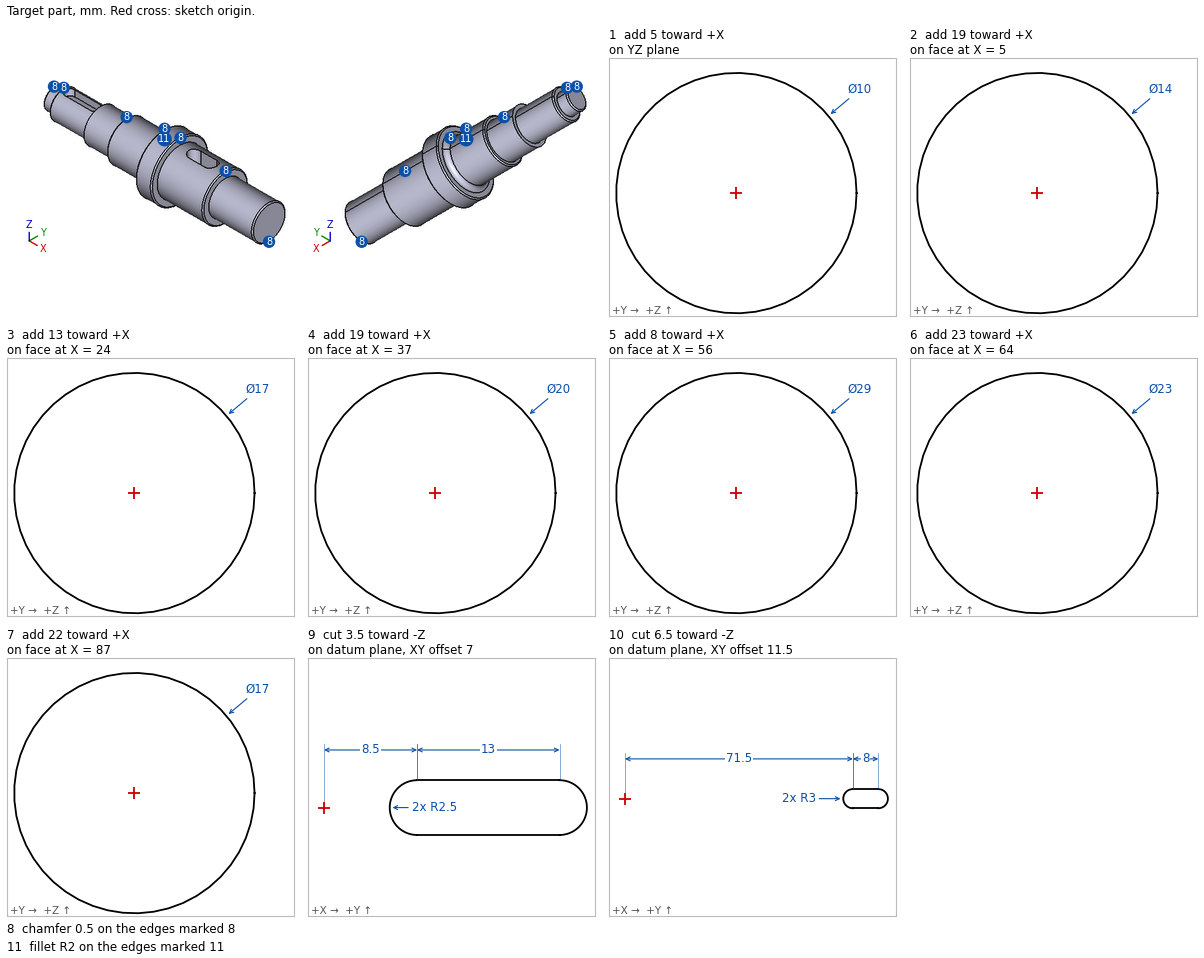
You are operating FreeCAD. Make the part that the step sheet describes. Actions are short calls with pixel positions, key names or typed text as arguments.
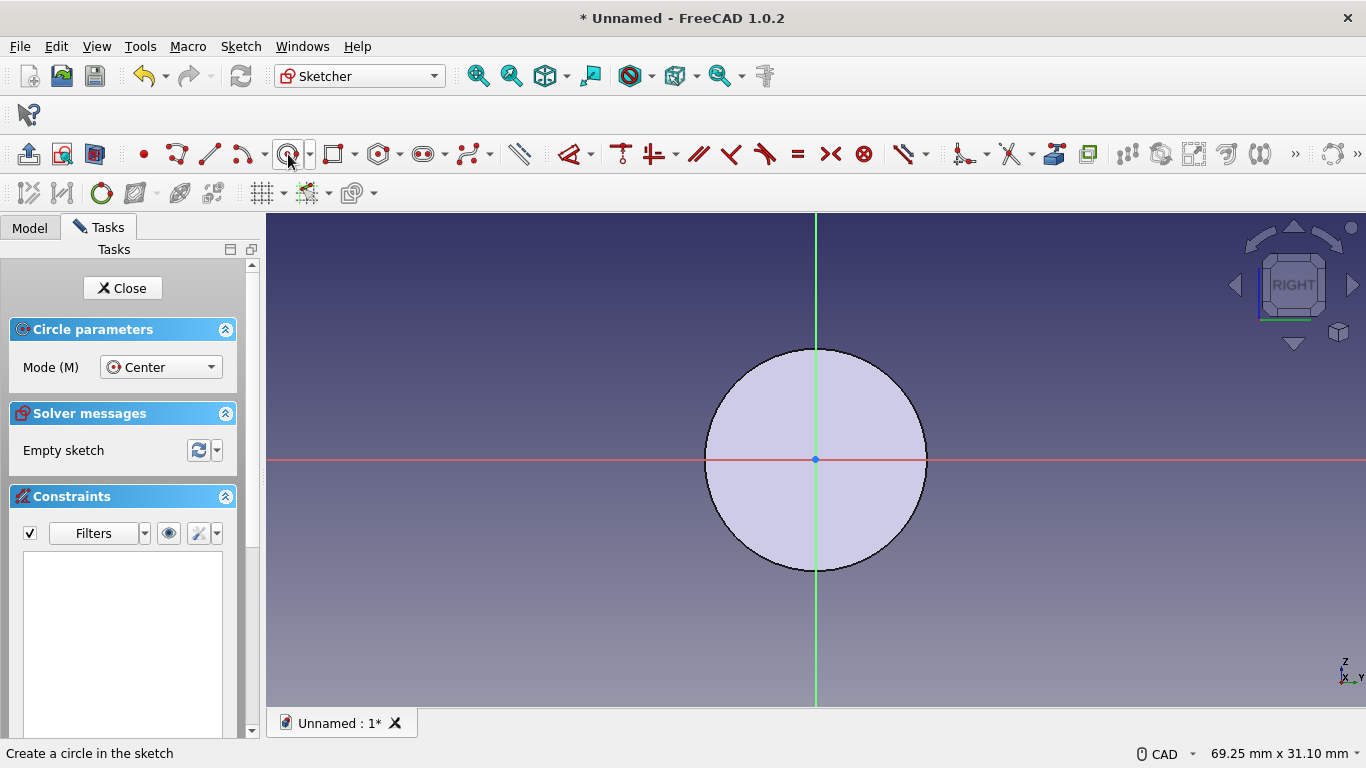
click(816, 460)
move(911, 365)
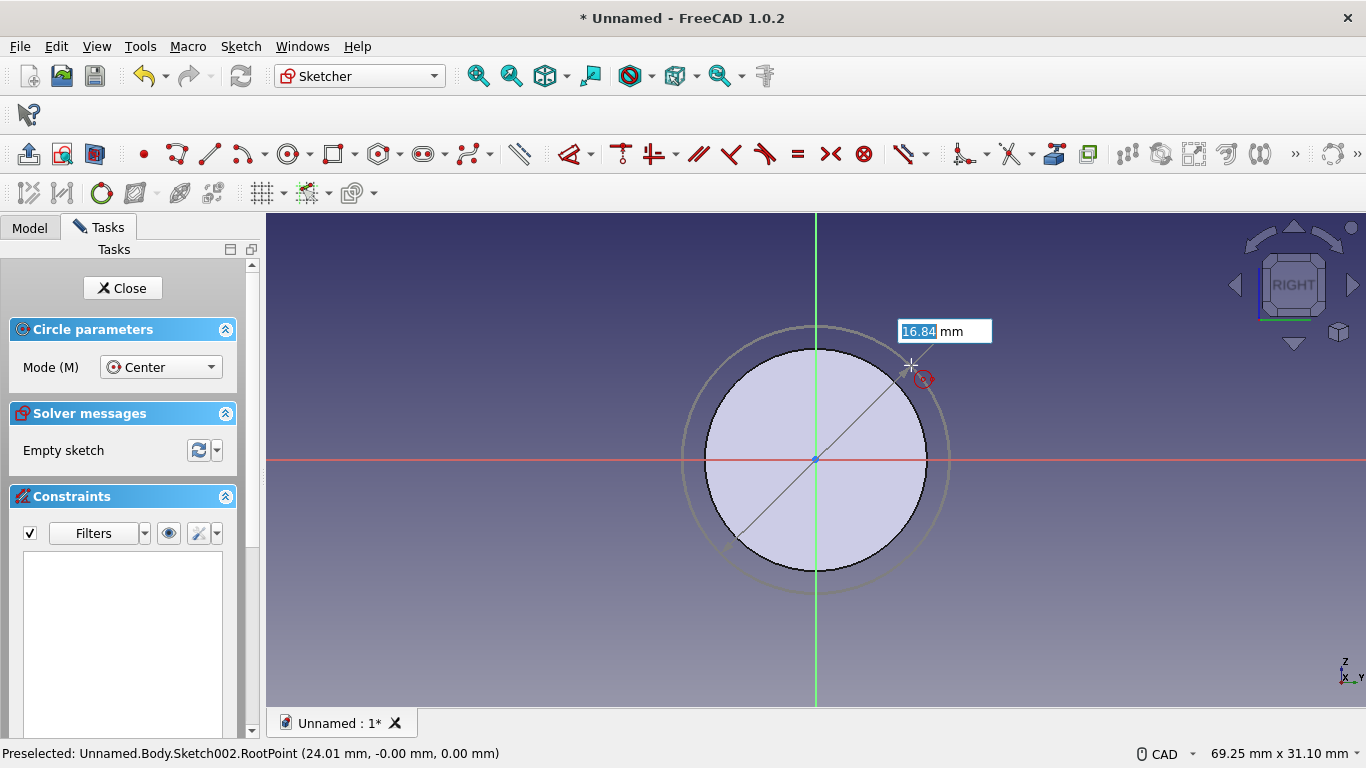
text(17)
key(Return)
key(Escape)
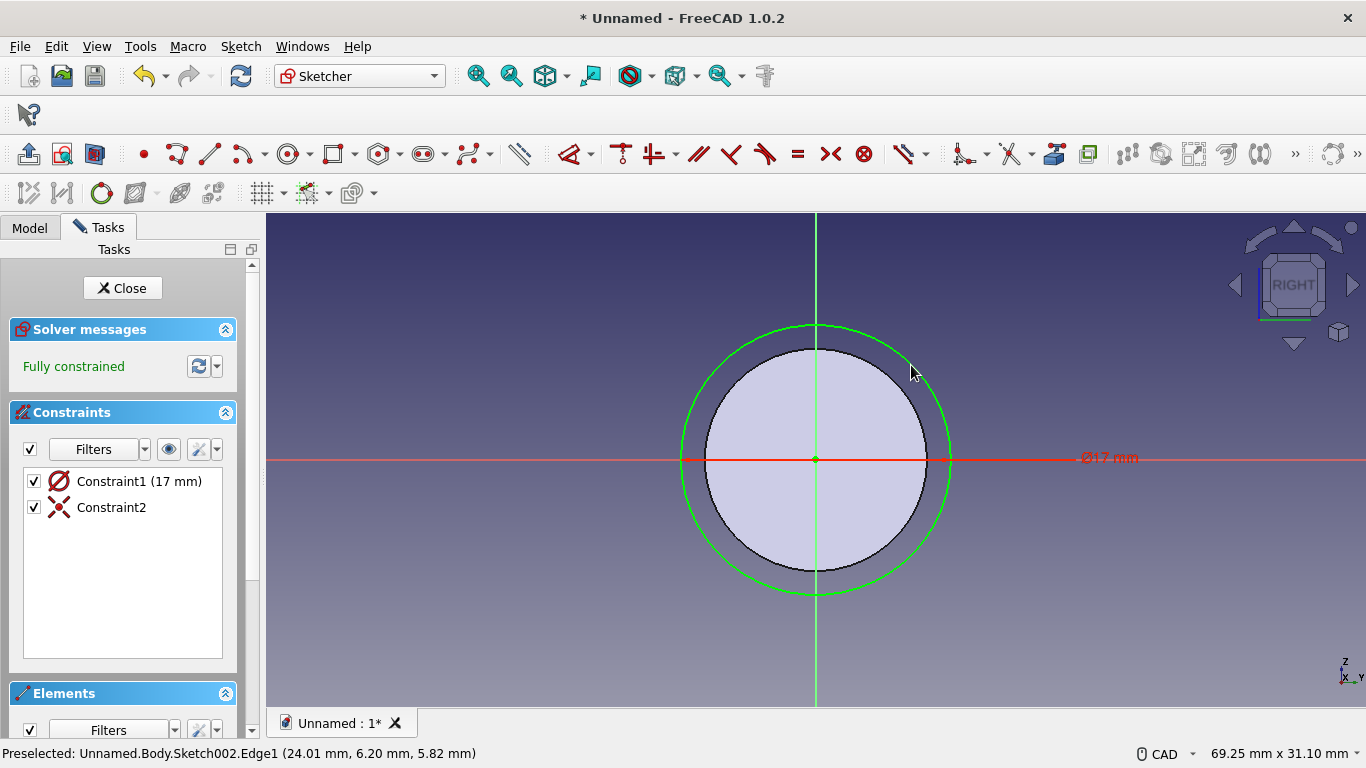
click(123, 288)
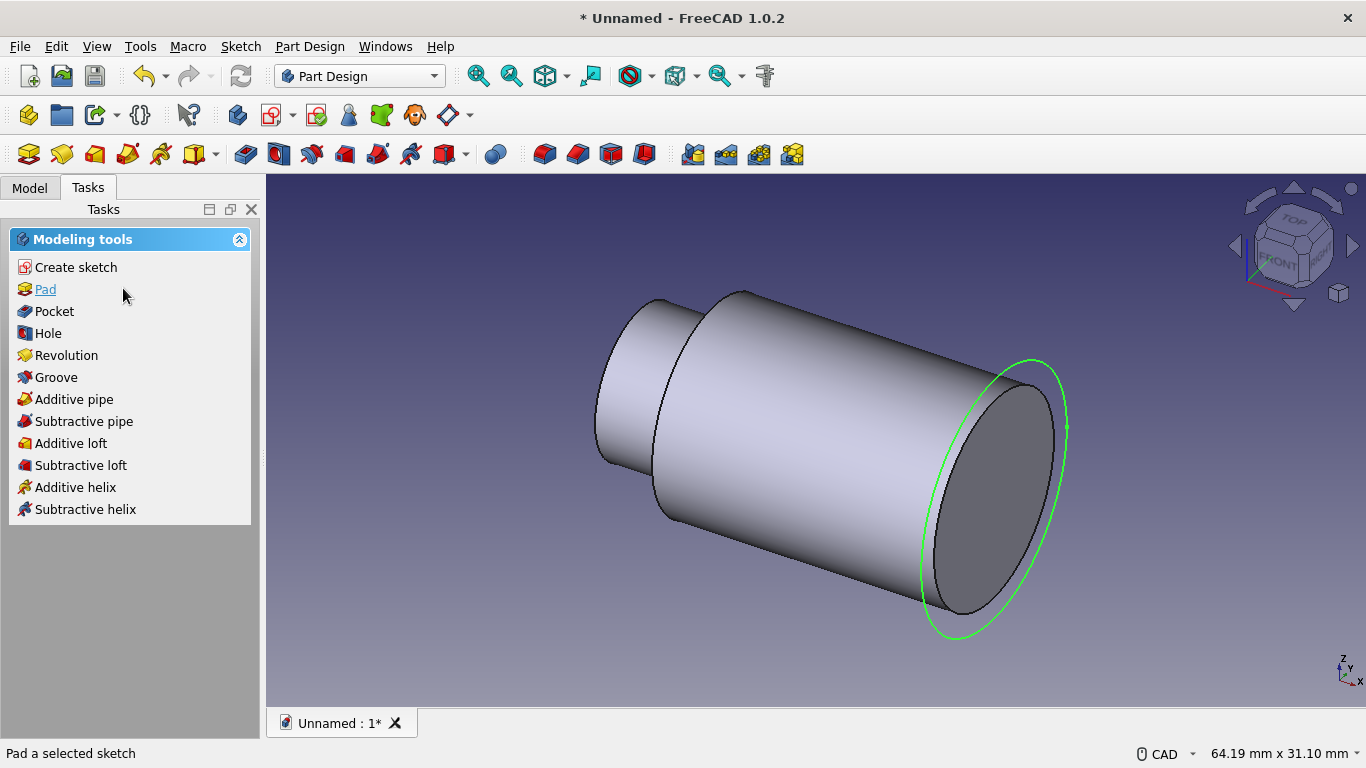
click(29, 154)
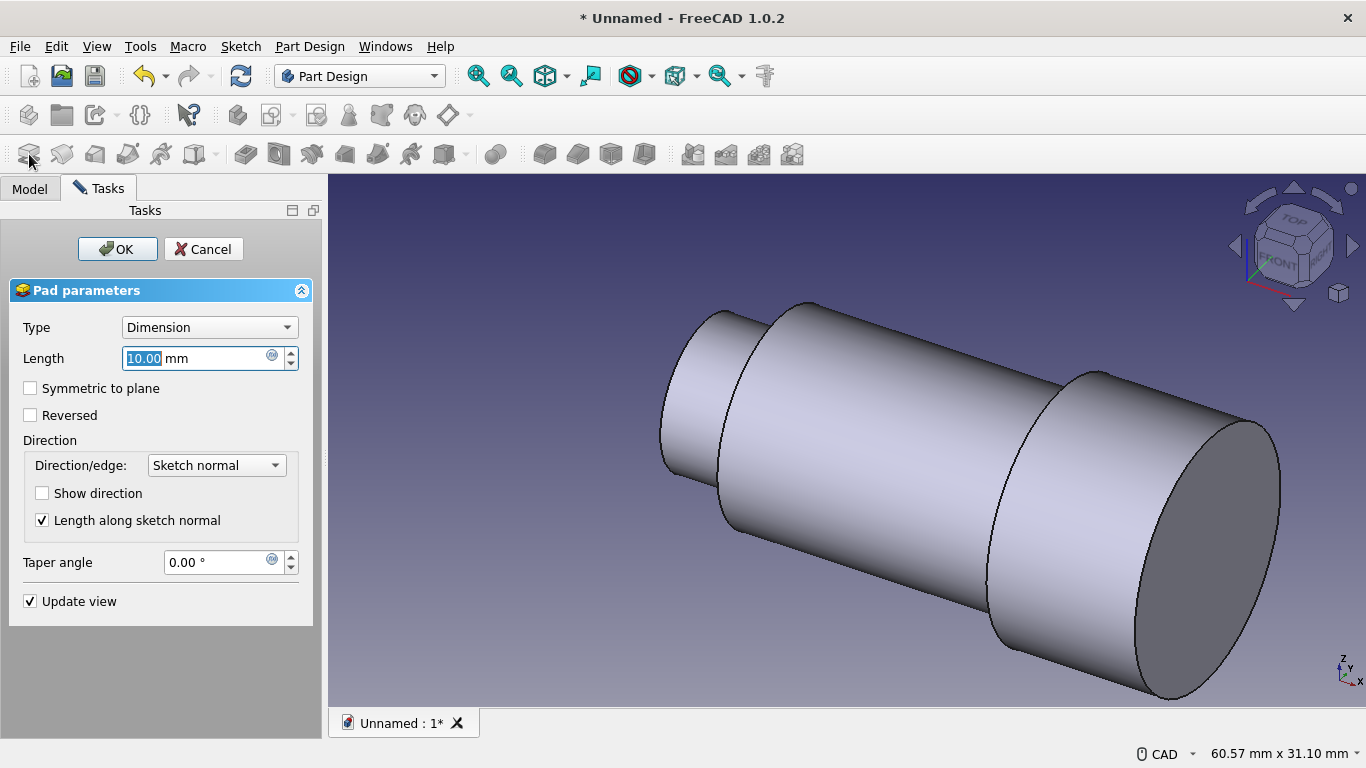
text(13)
key(Tab)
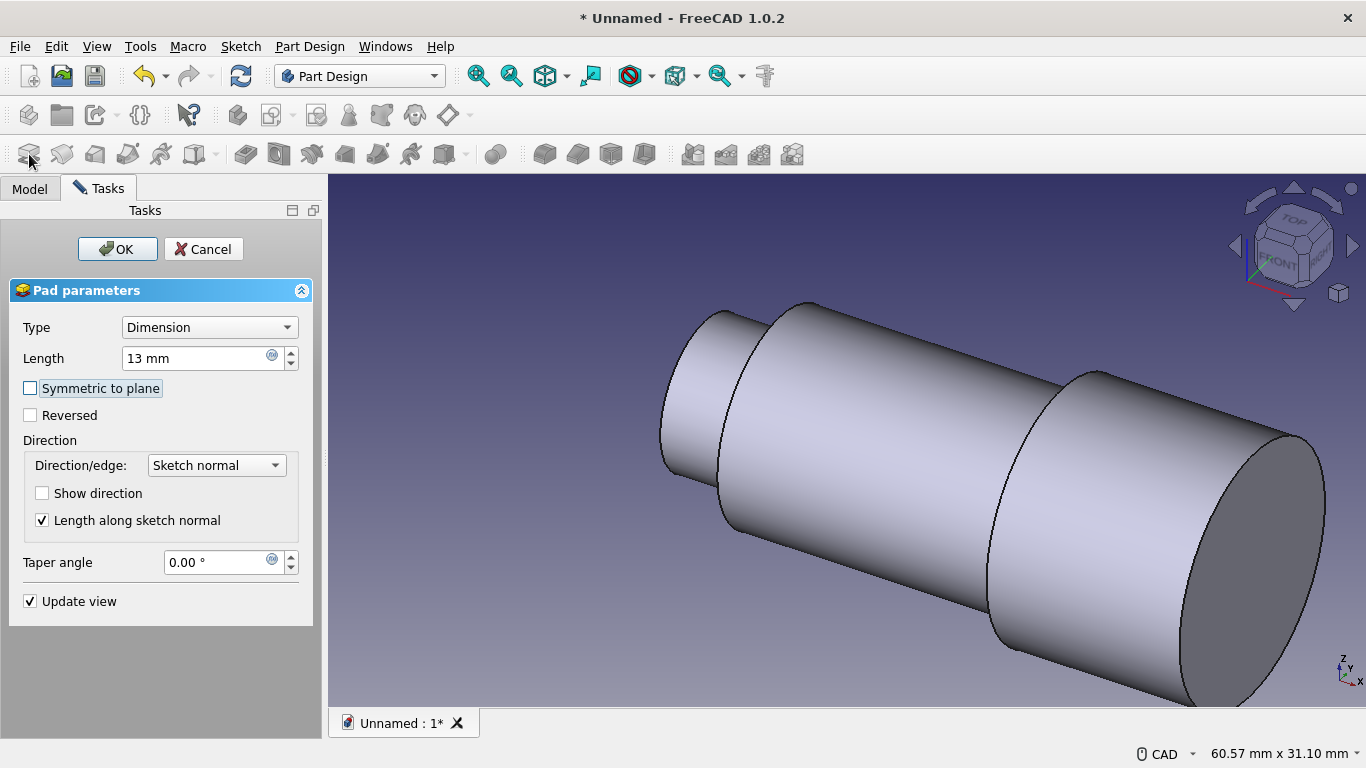
click(118, 249)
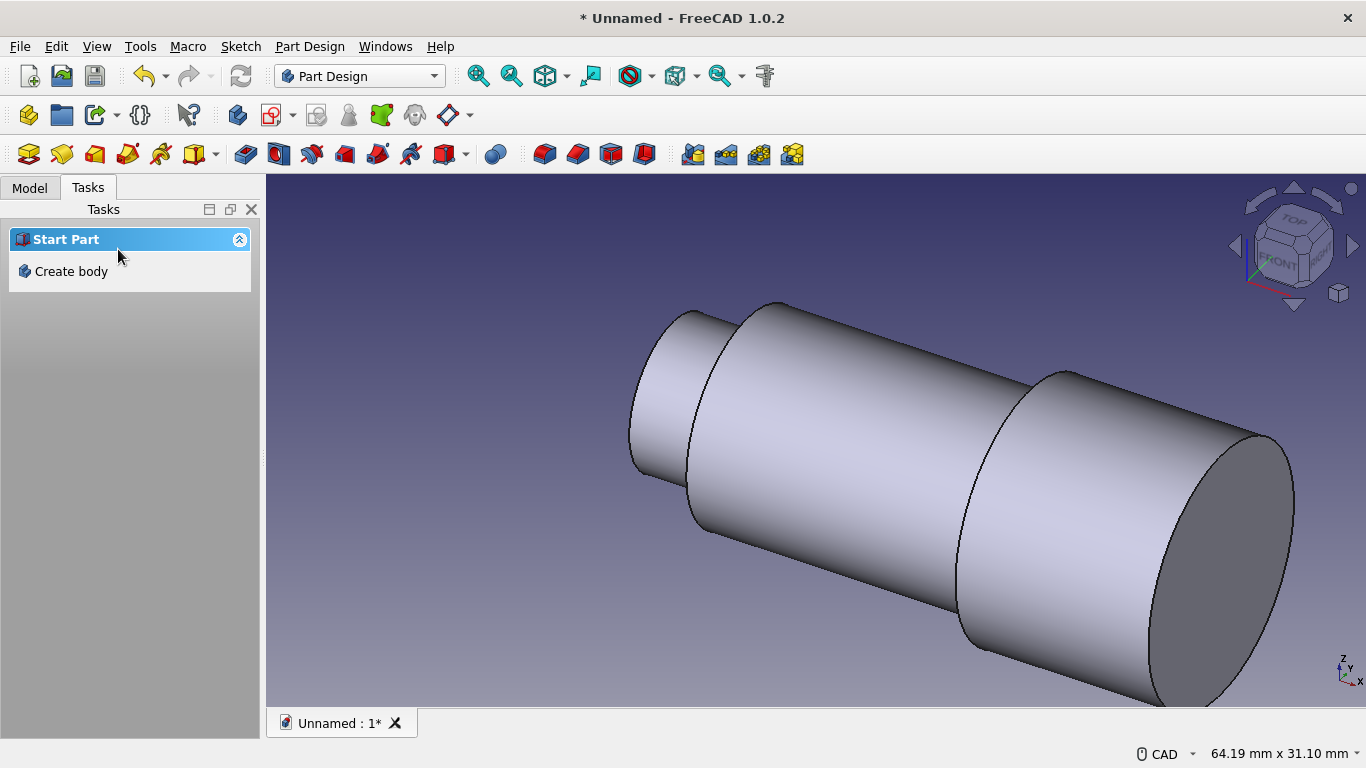
click(479, 76)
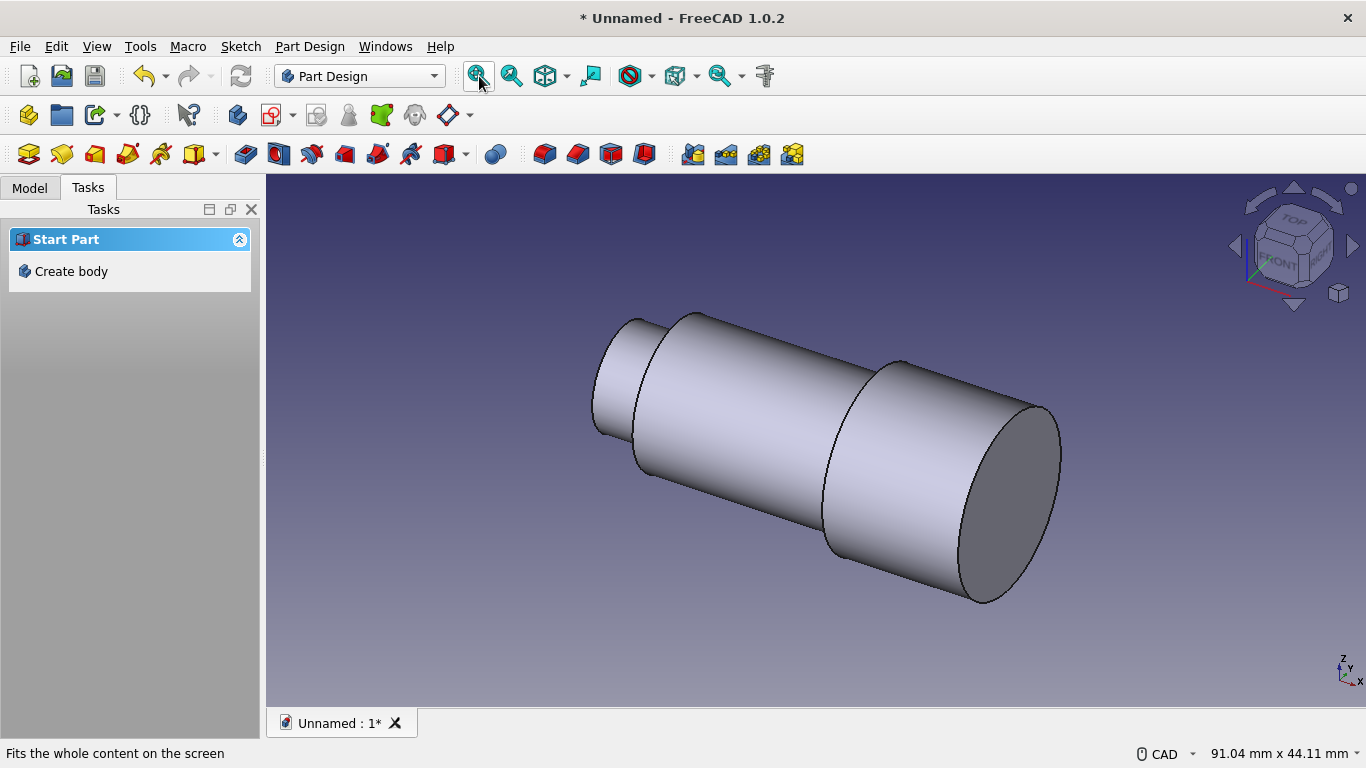
click(1010, 504)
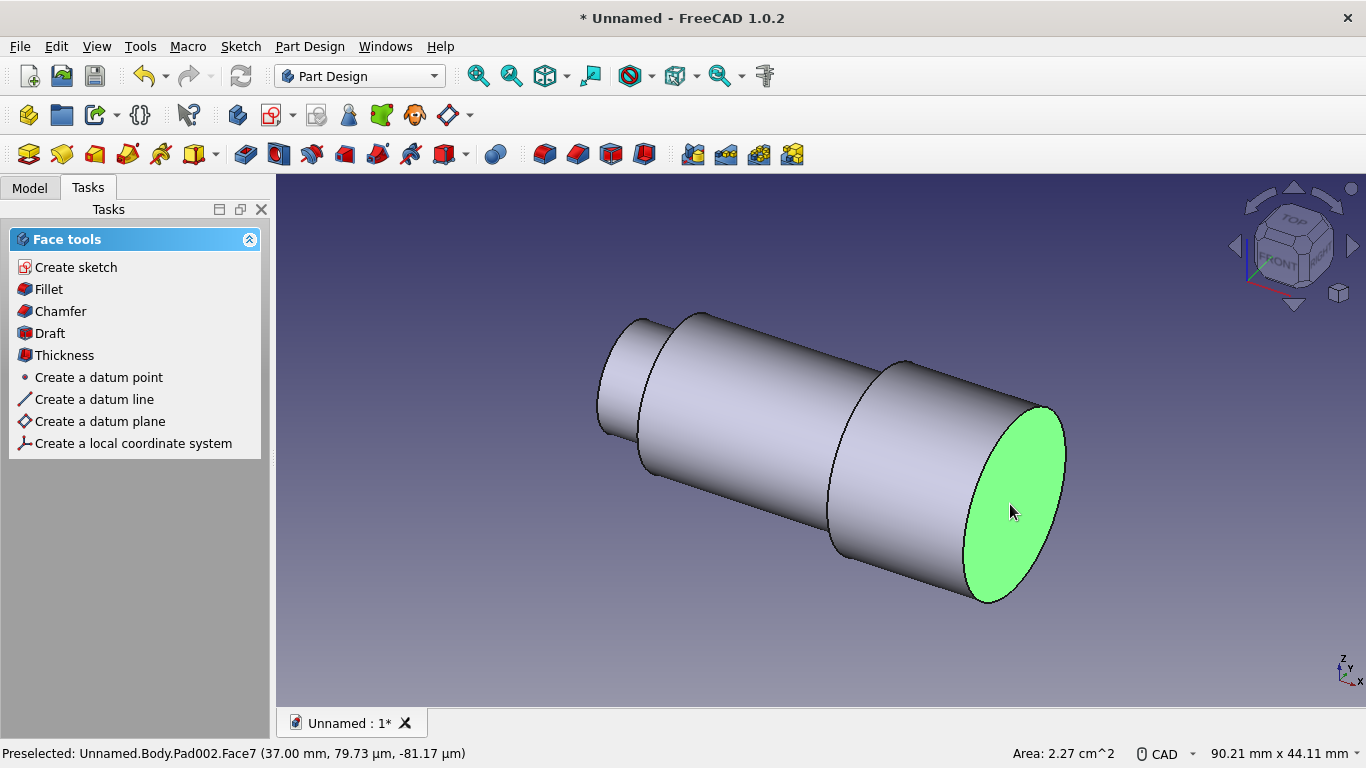
click(270, 116)